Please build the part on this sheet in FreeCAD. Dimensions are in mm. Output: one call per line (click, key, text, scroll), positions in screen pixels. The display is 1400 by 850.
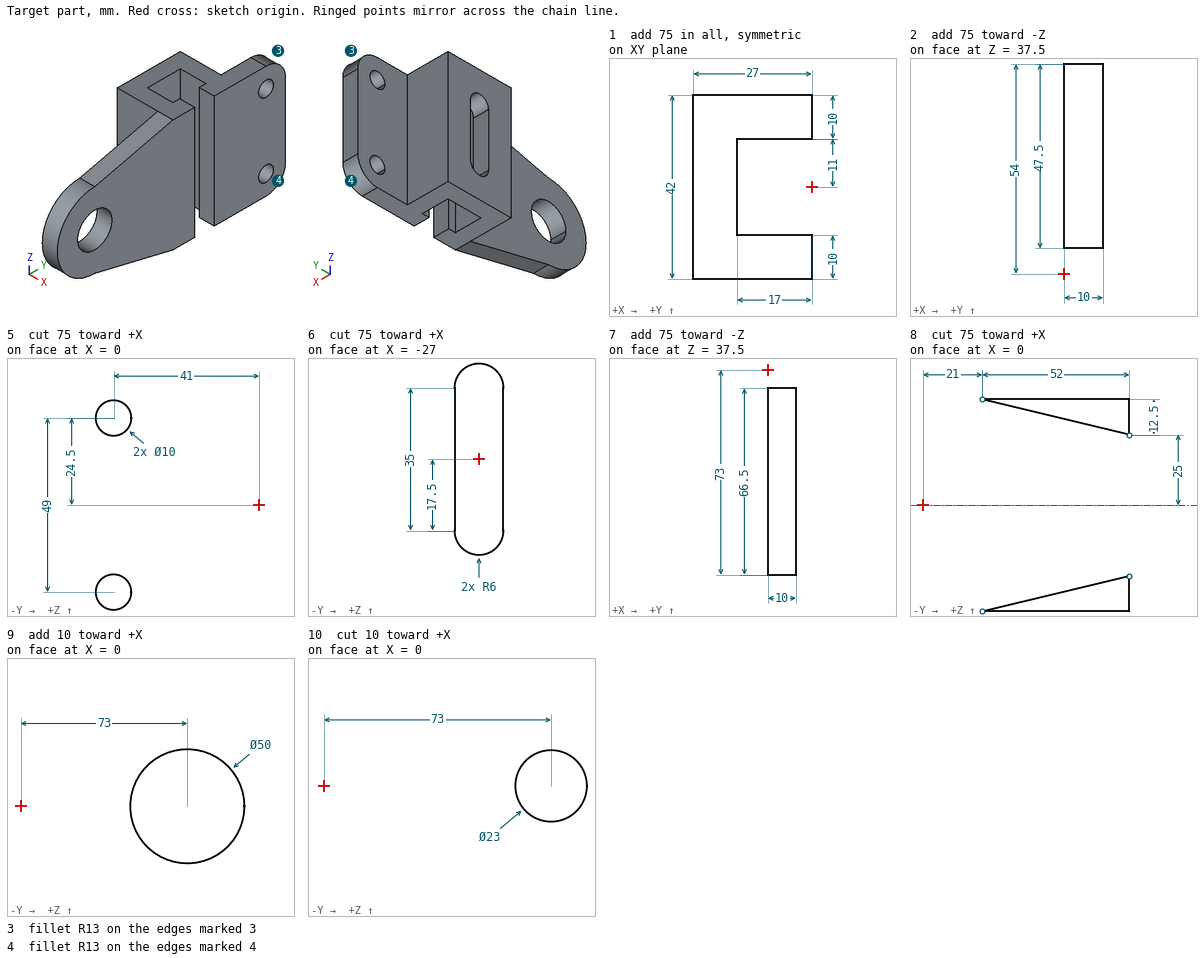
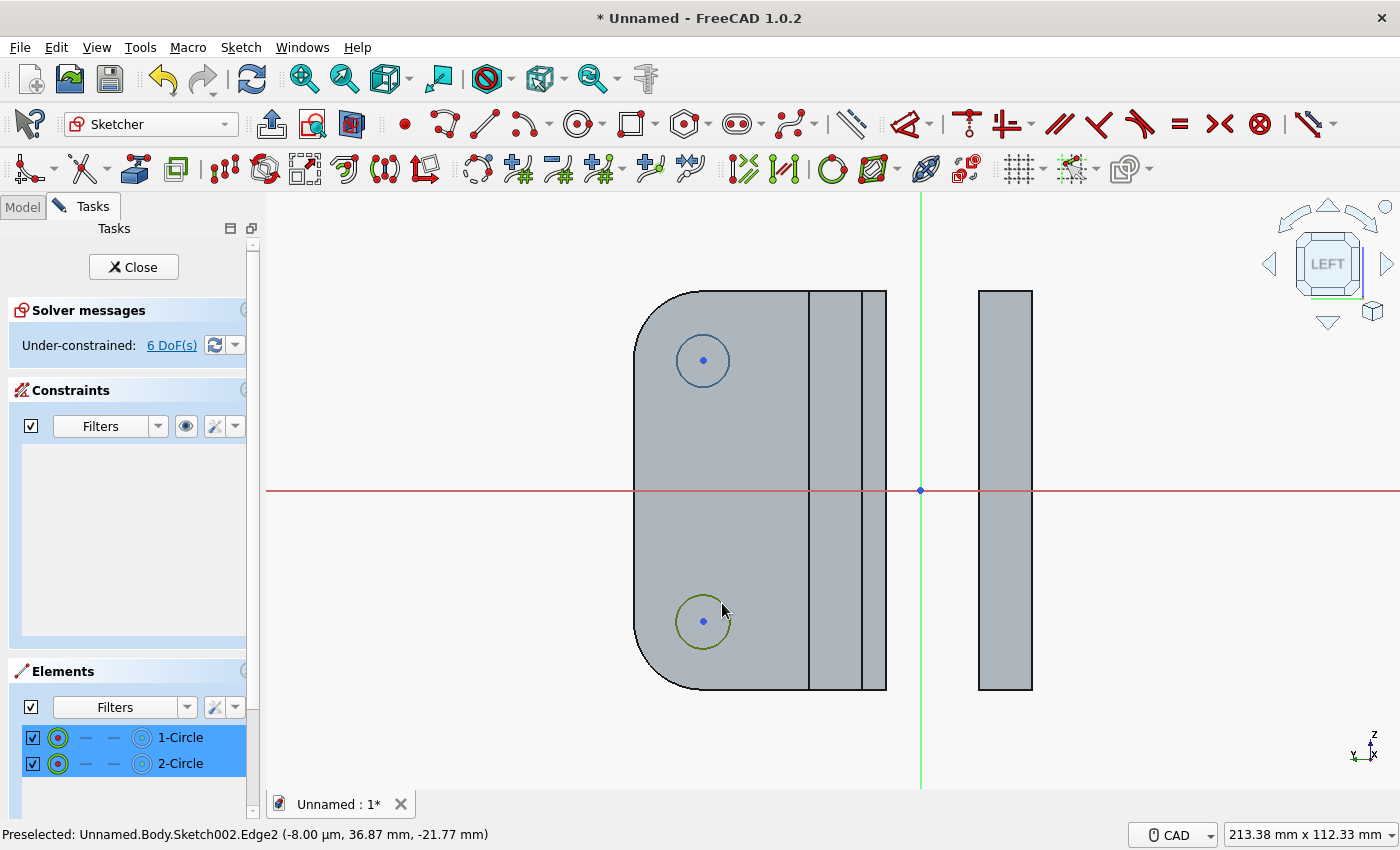
key(e)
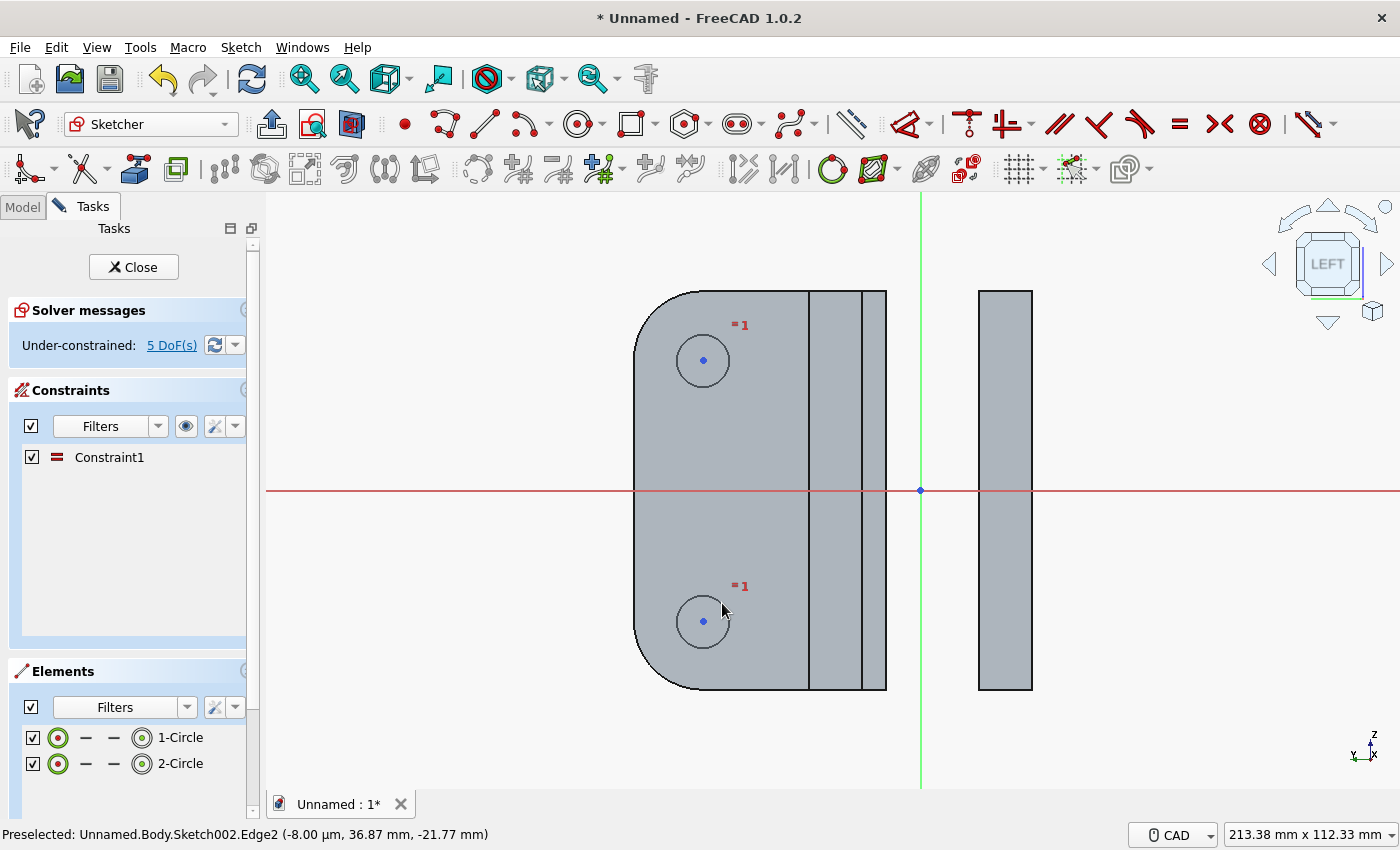
click(703, 361)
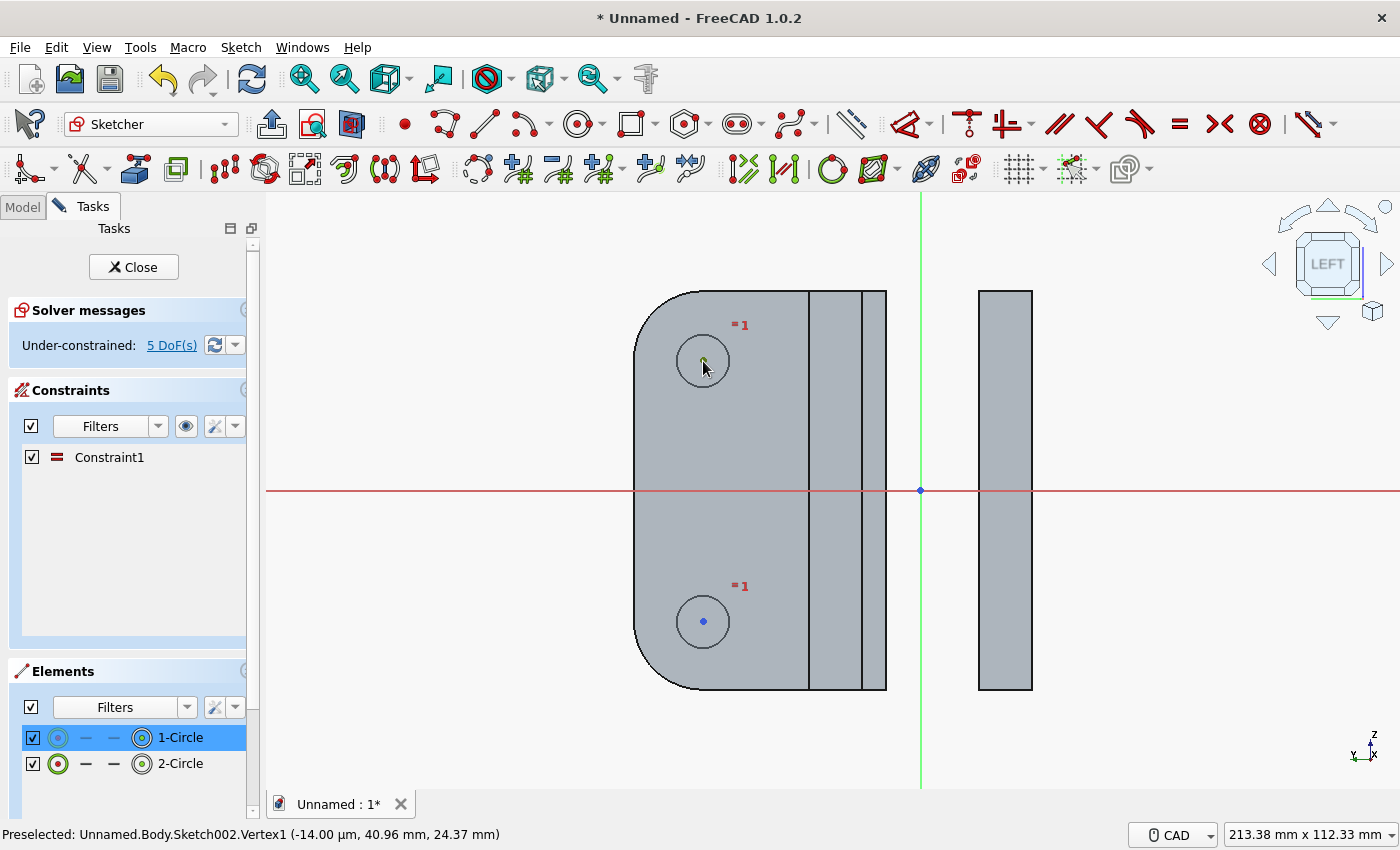
click(703, 622)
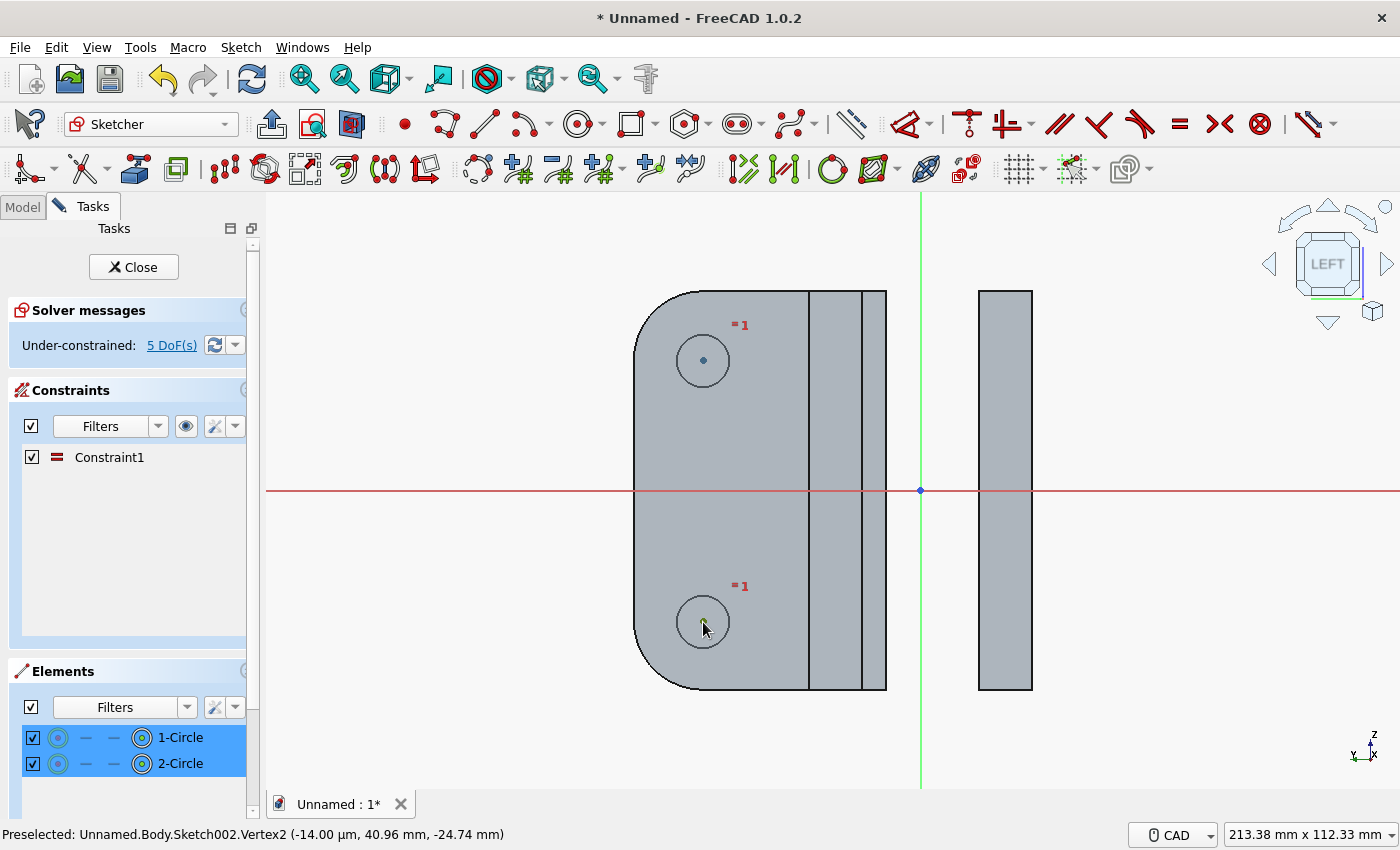
key(v)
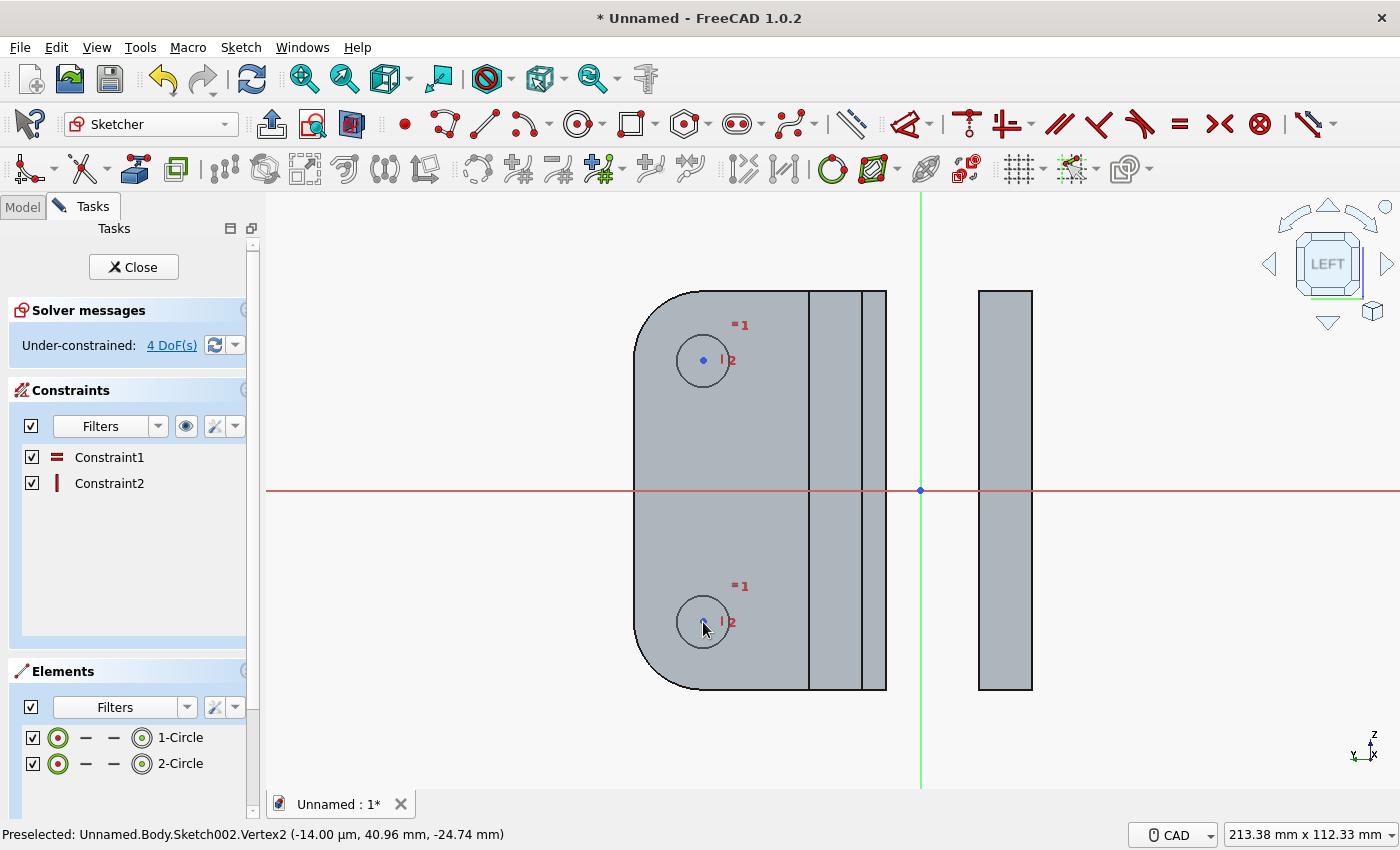
key(d)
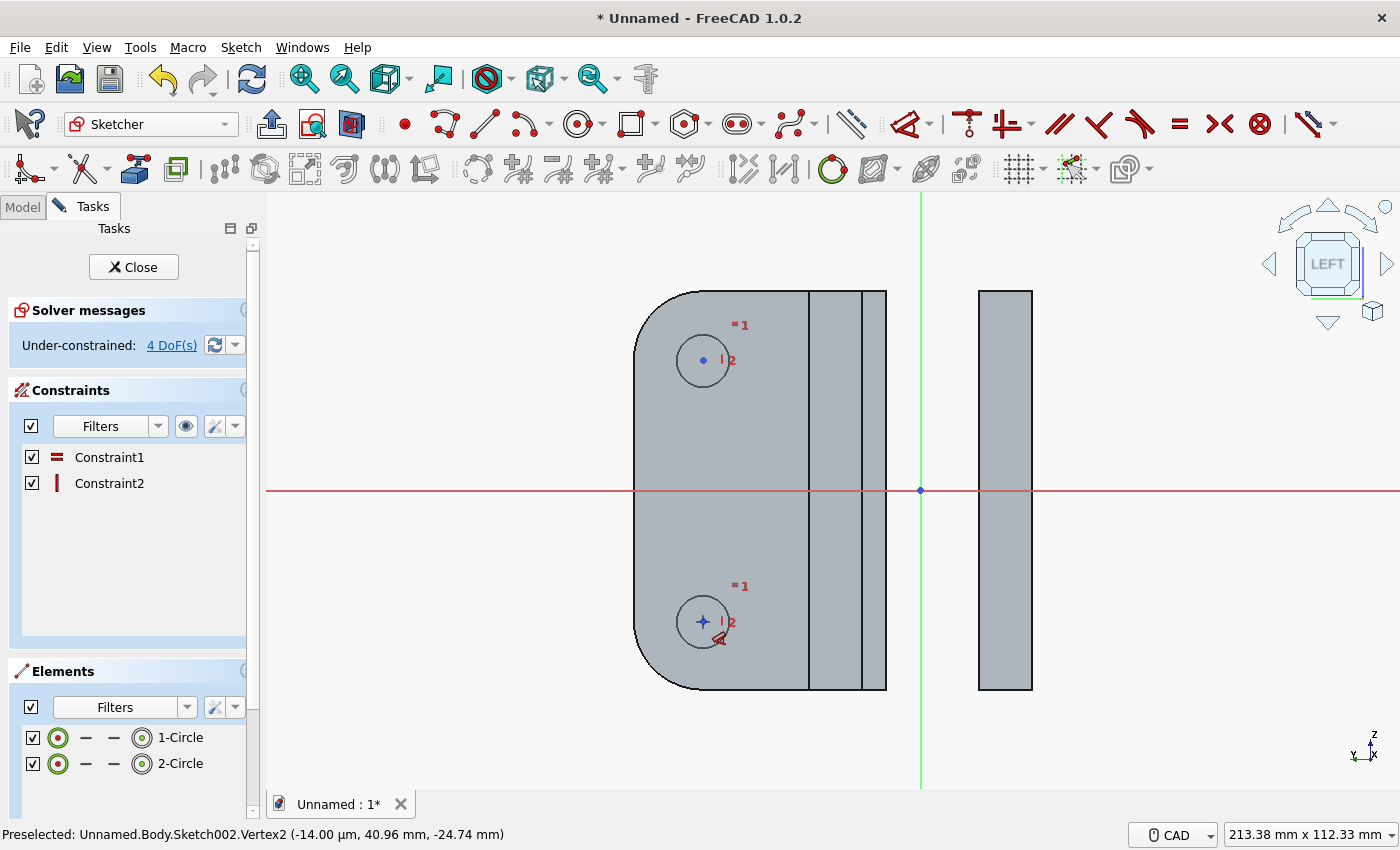
click(721, 342)
click(743, 319)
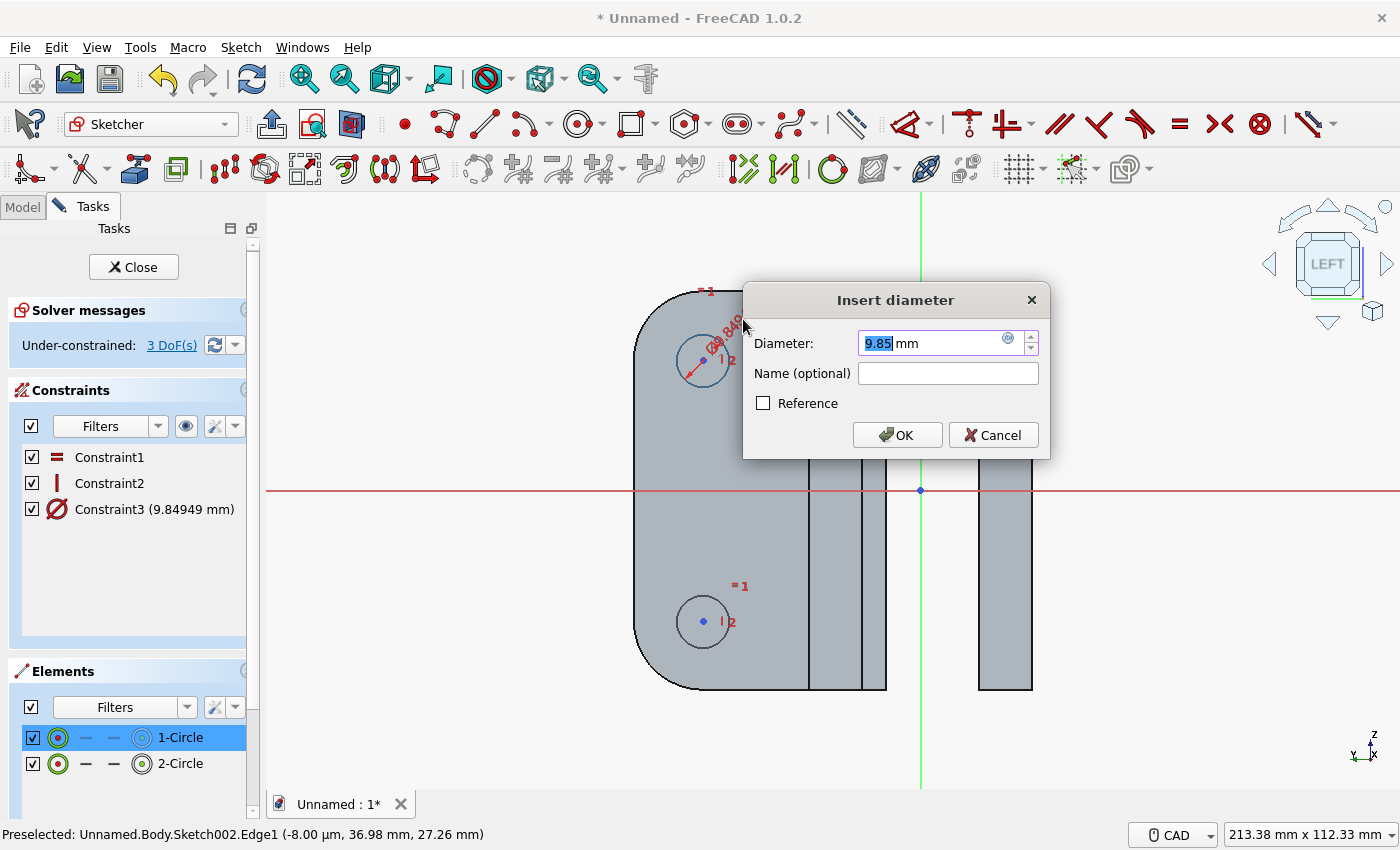
text(10)
key(Return)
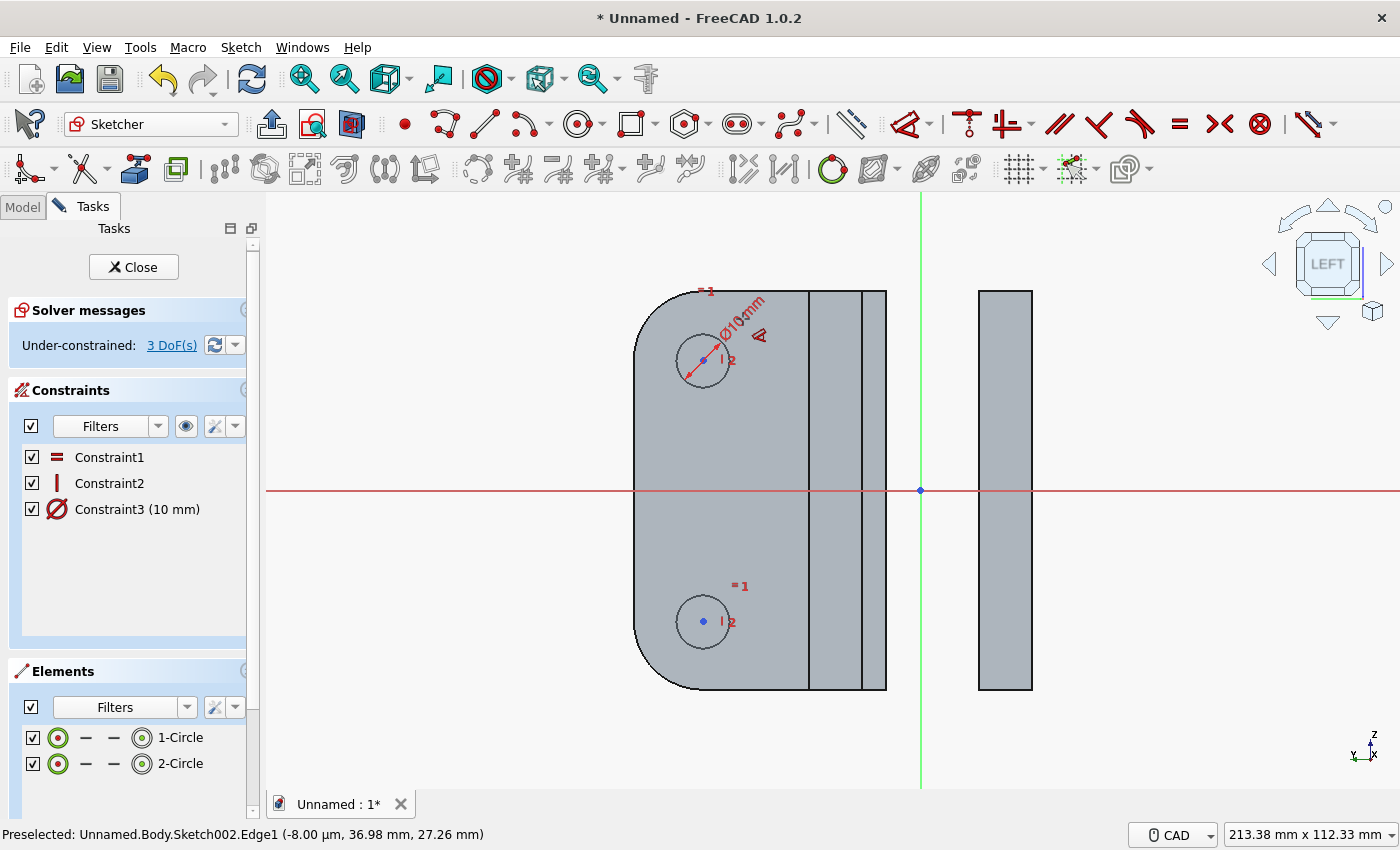
click(703, 361)
click(862, 327)